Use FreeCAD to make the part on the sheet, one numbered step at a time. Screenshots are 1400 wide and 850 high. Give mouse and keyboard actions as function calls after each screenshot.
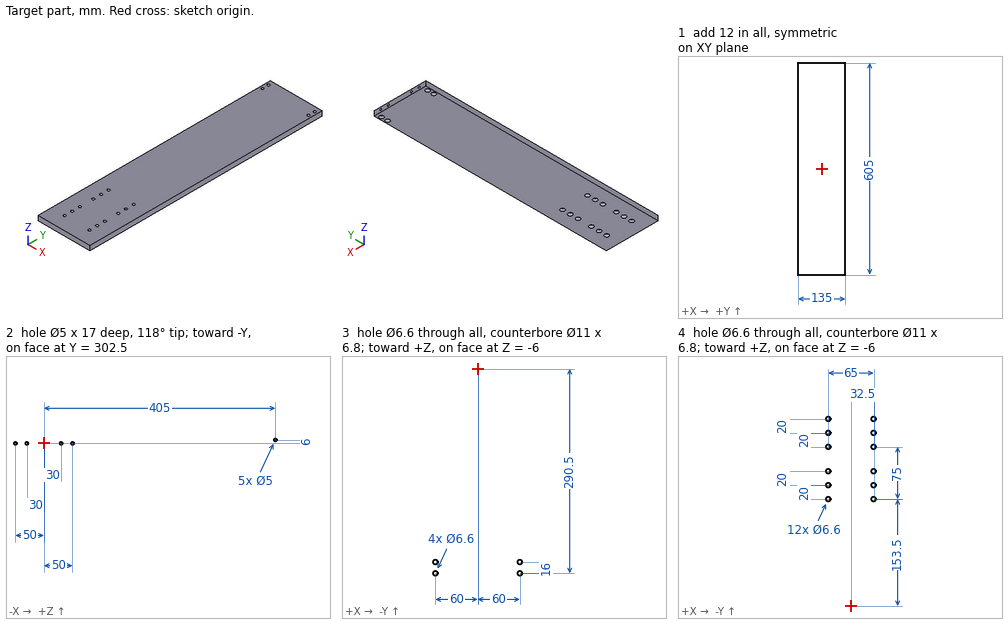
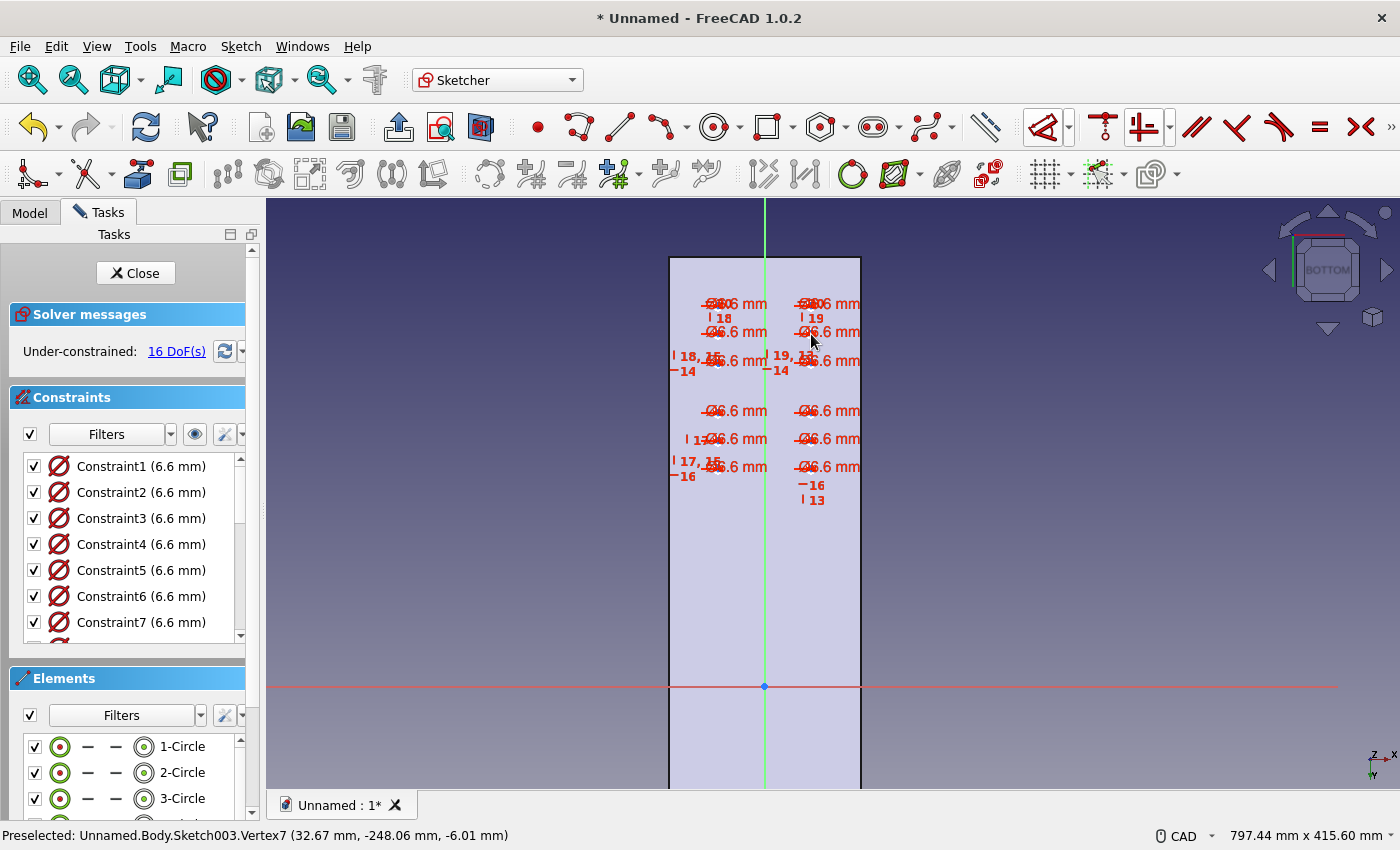
click(811, 469)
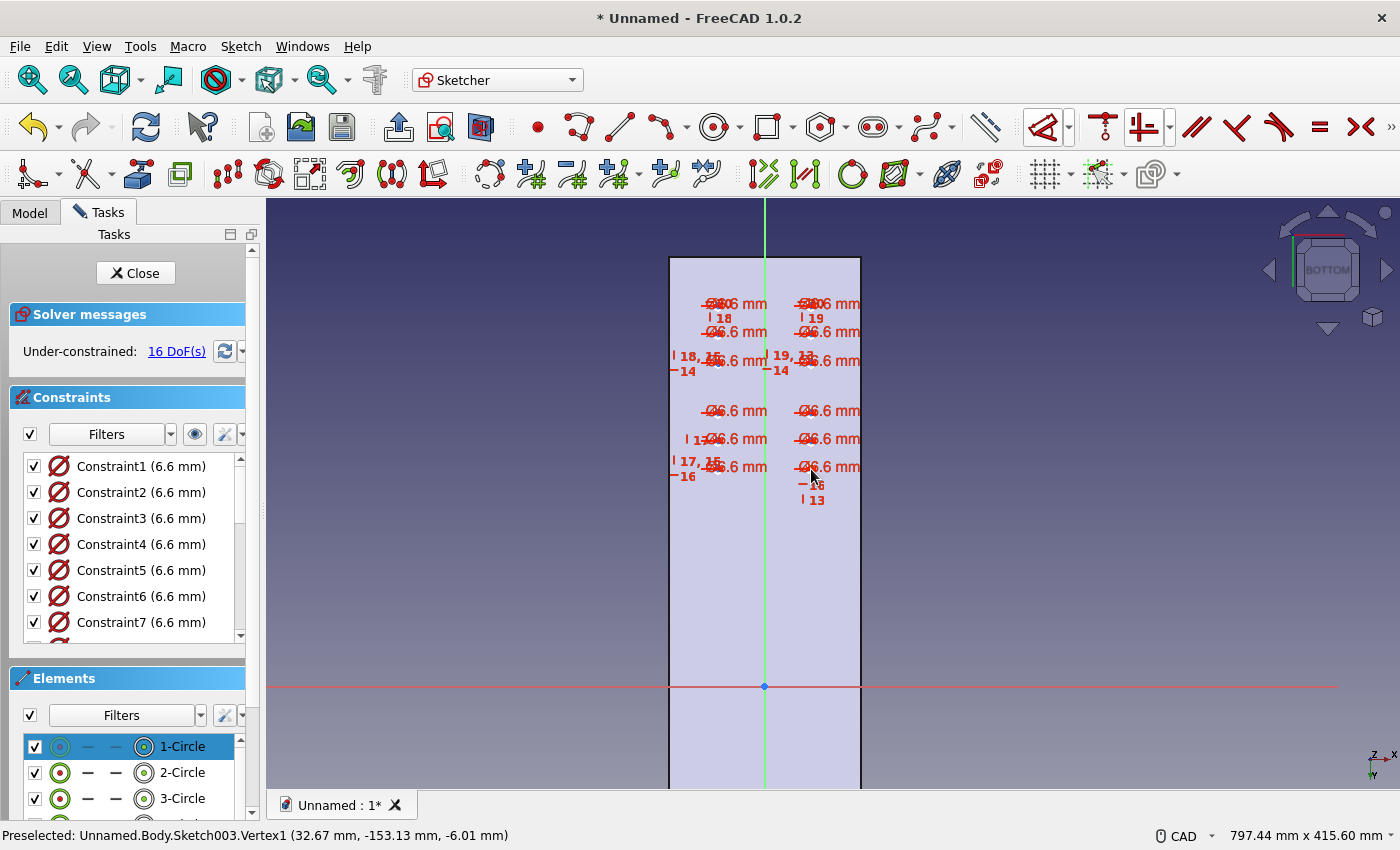
click(811, 441)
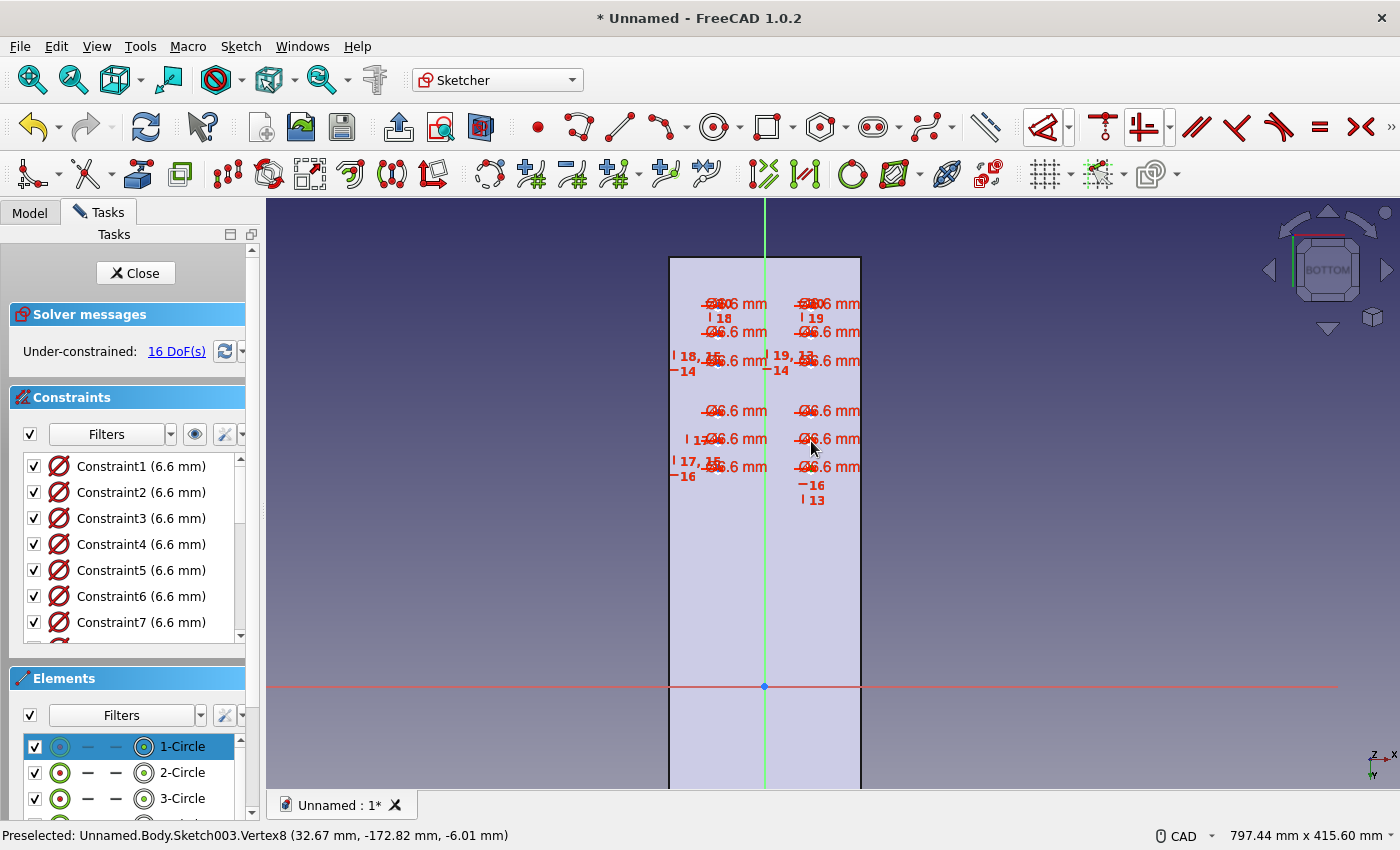
key(v)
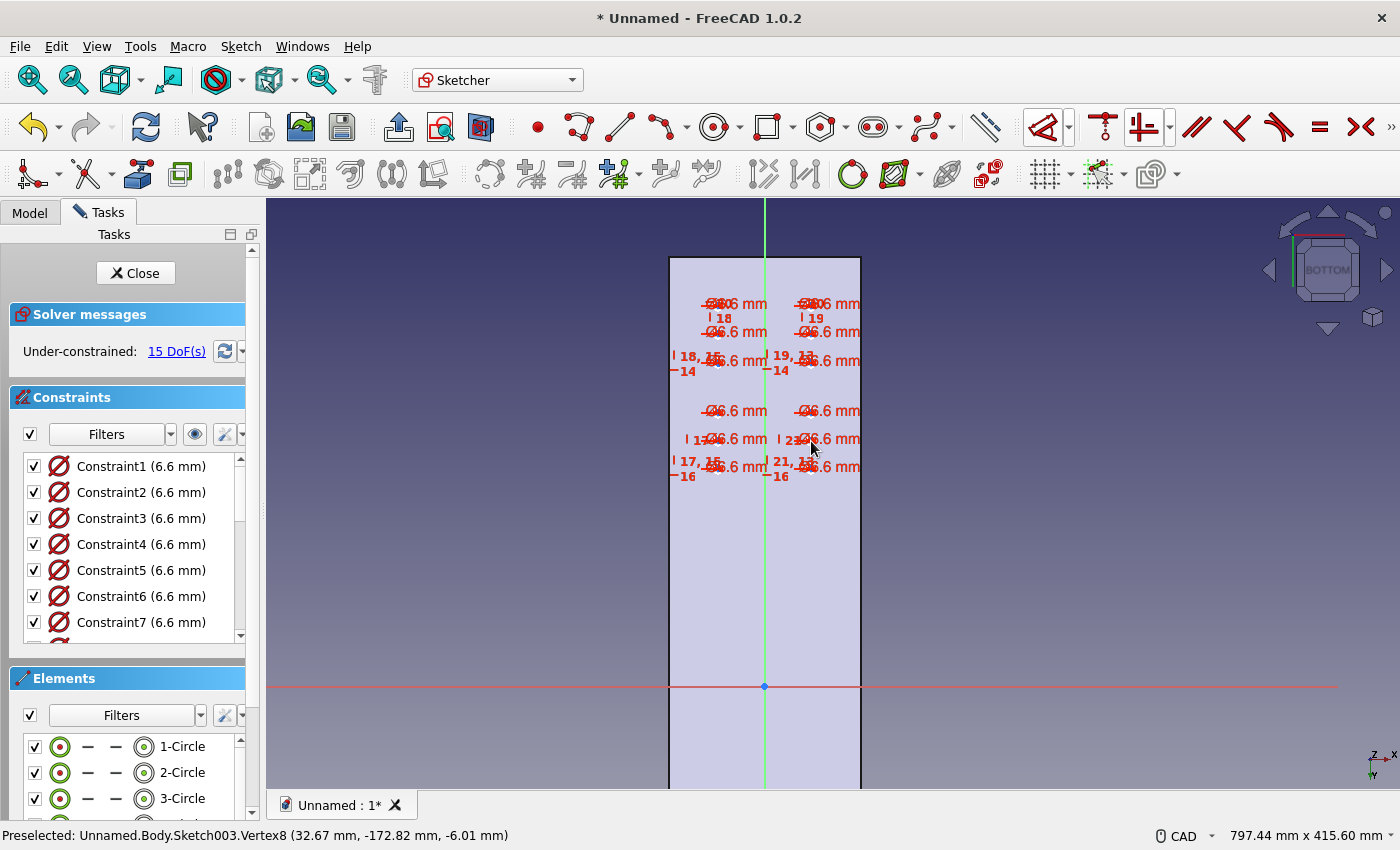
click(718, 441)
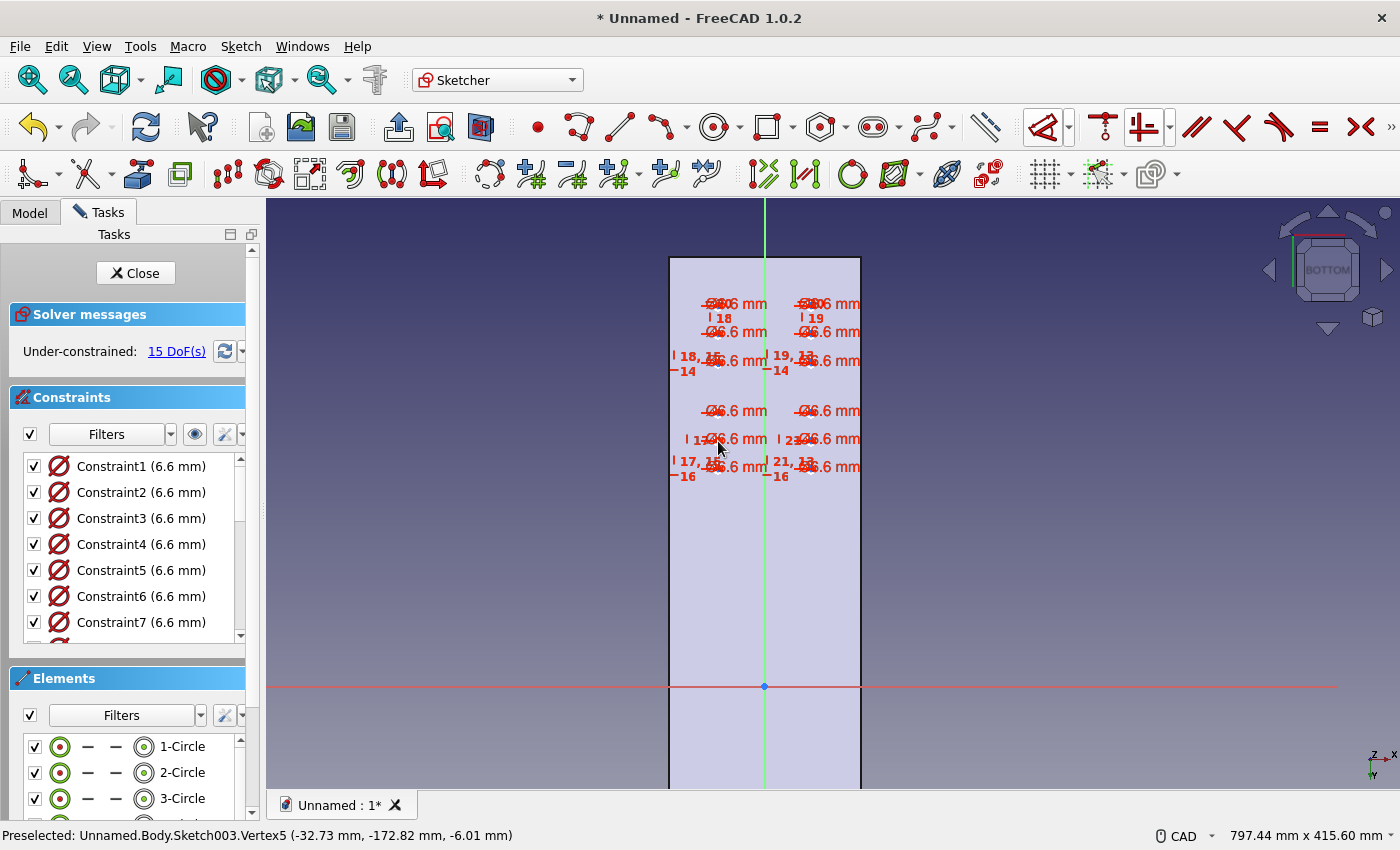
click(811, 441)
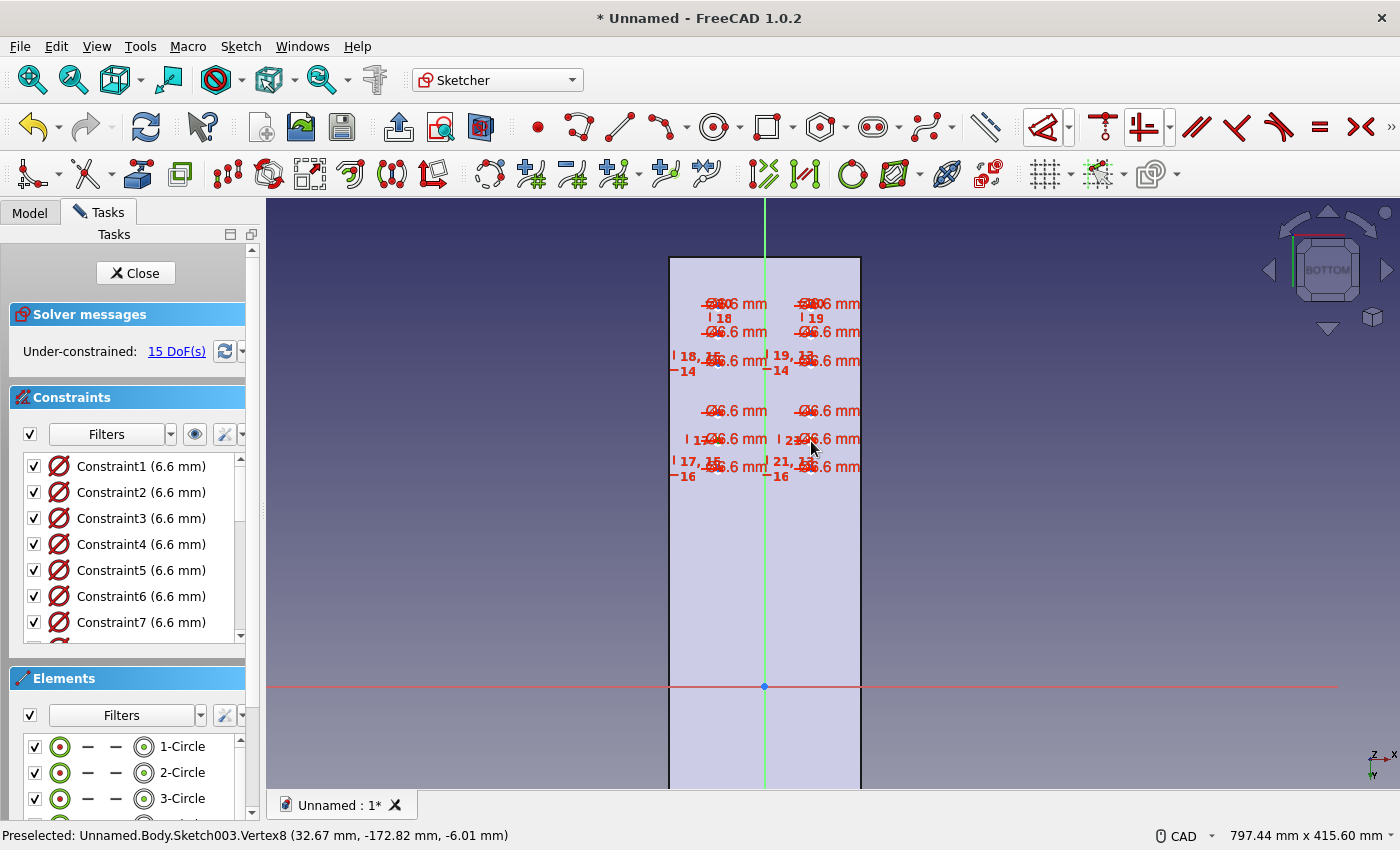
key(h)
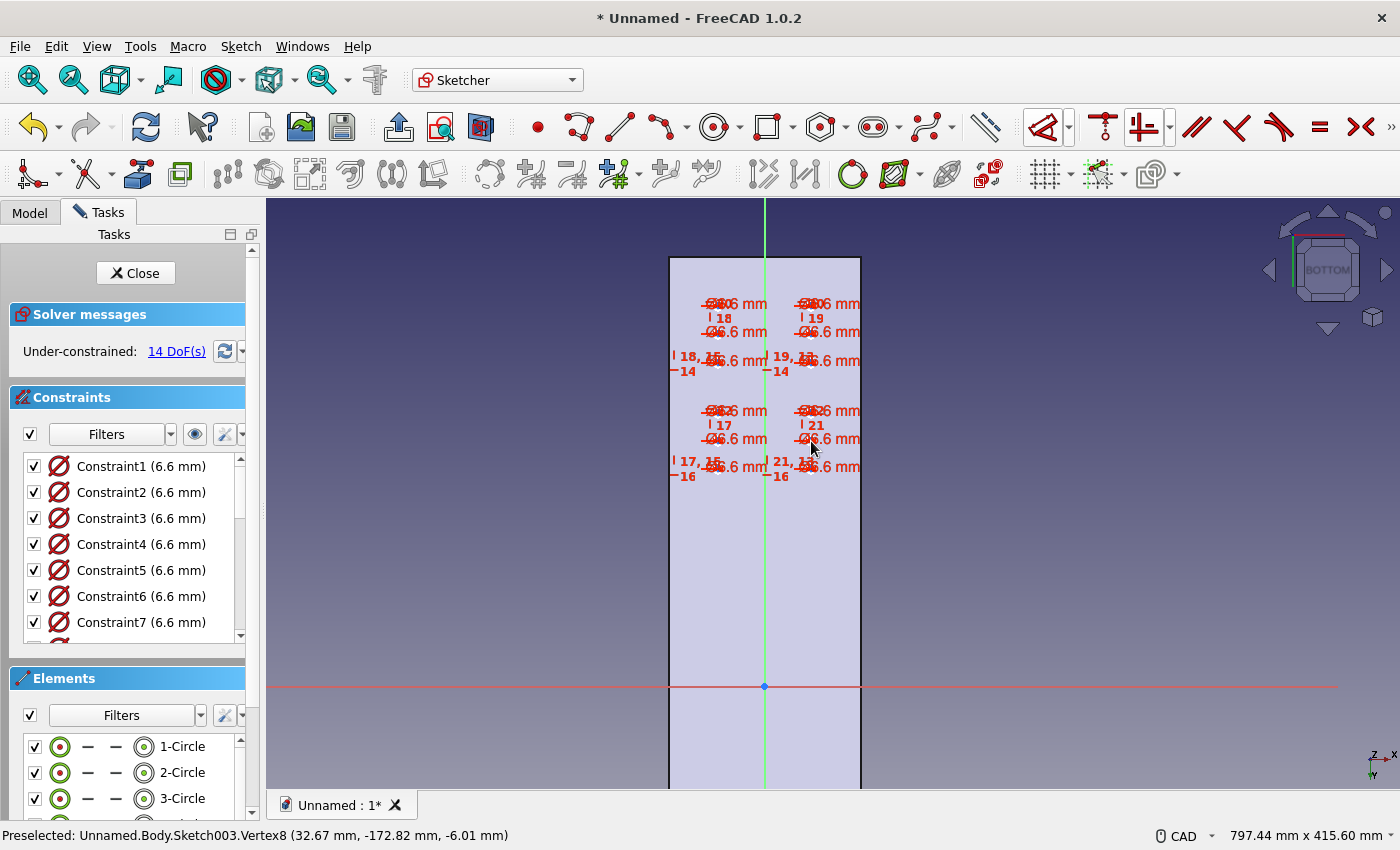
click(718, 334)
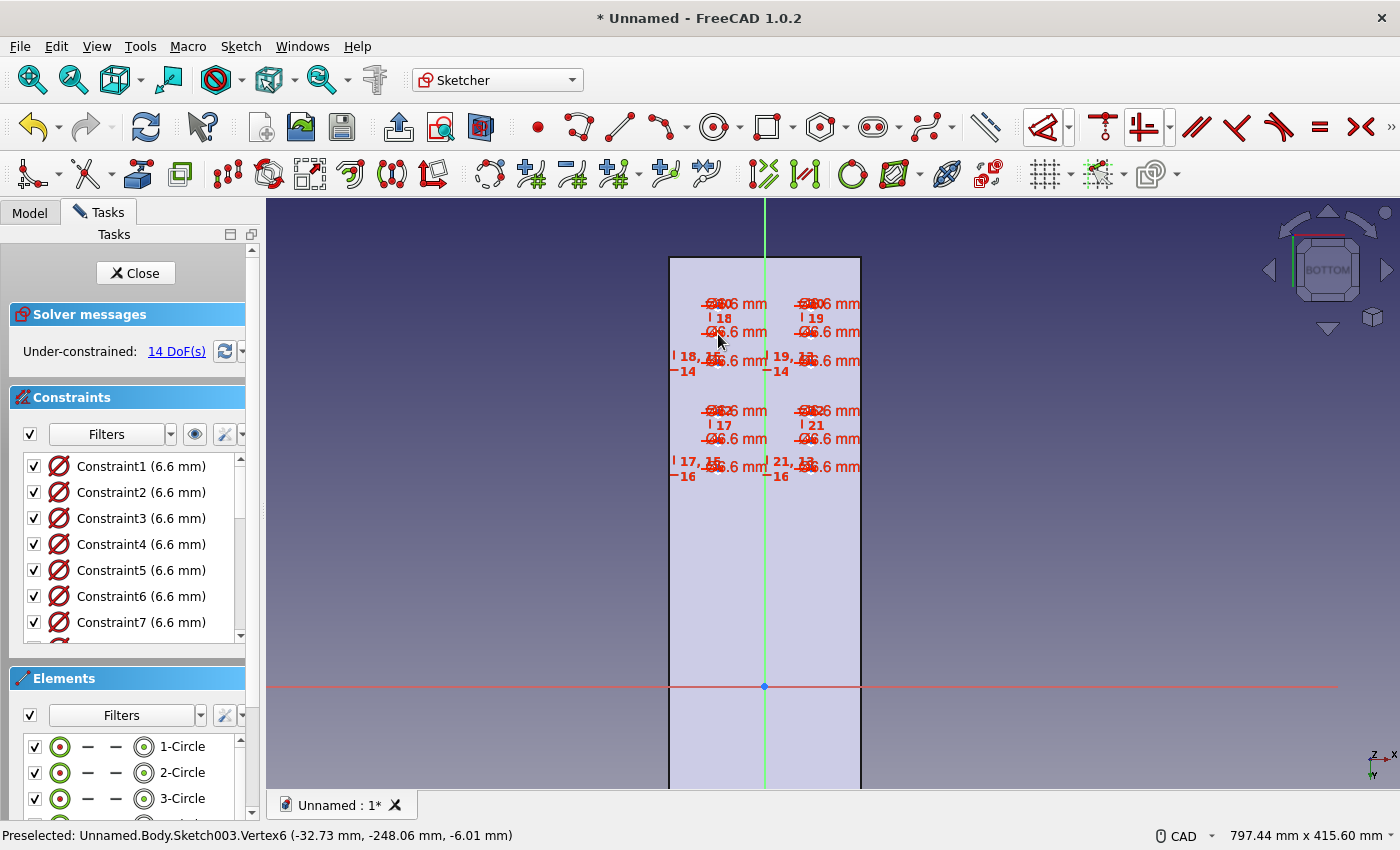
click(718, 306)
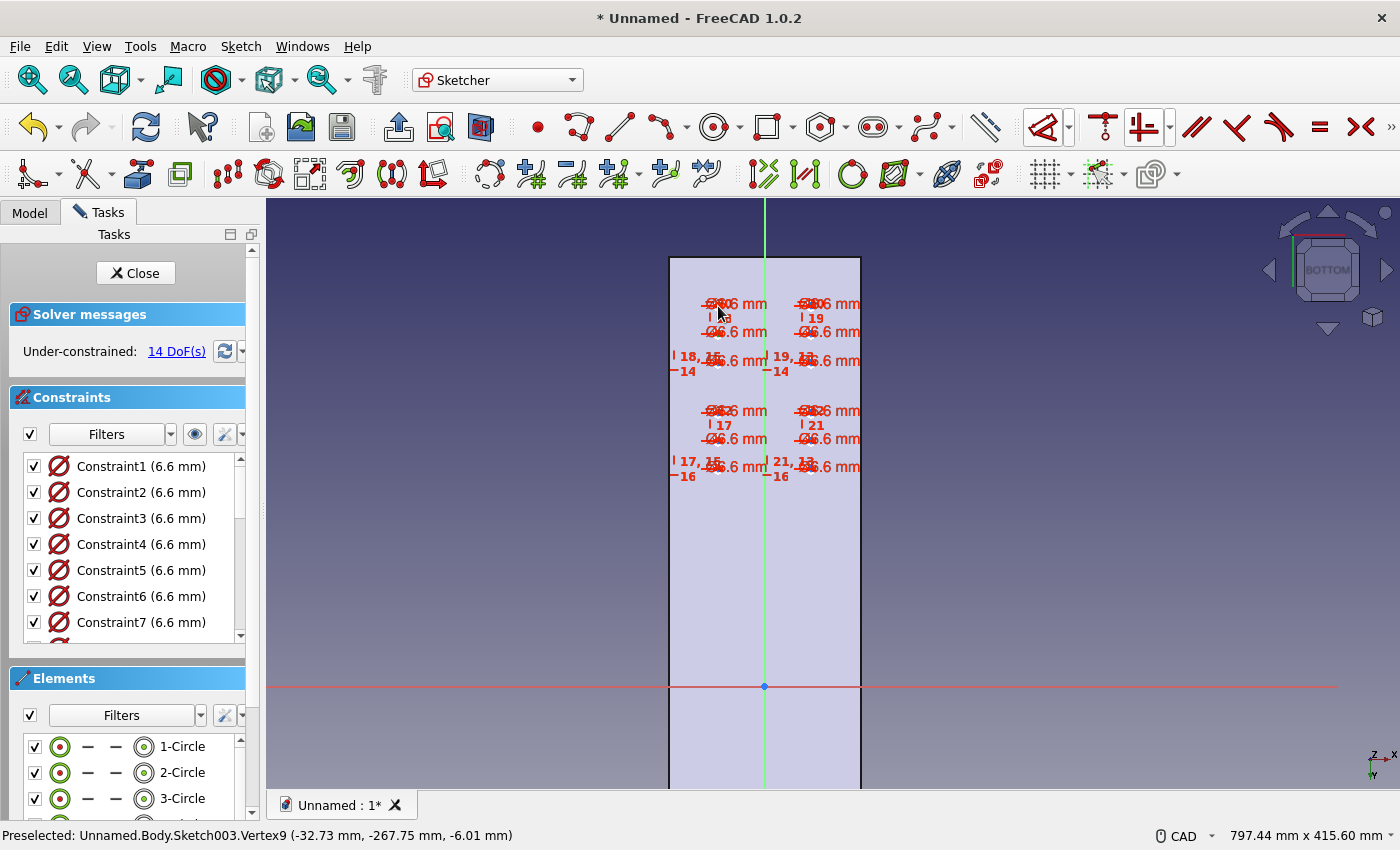
click(1170, 128)